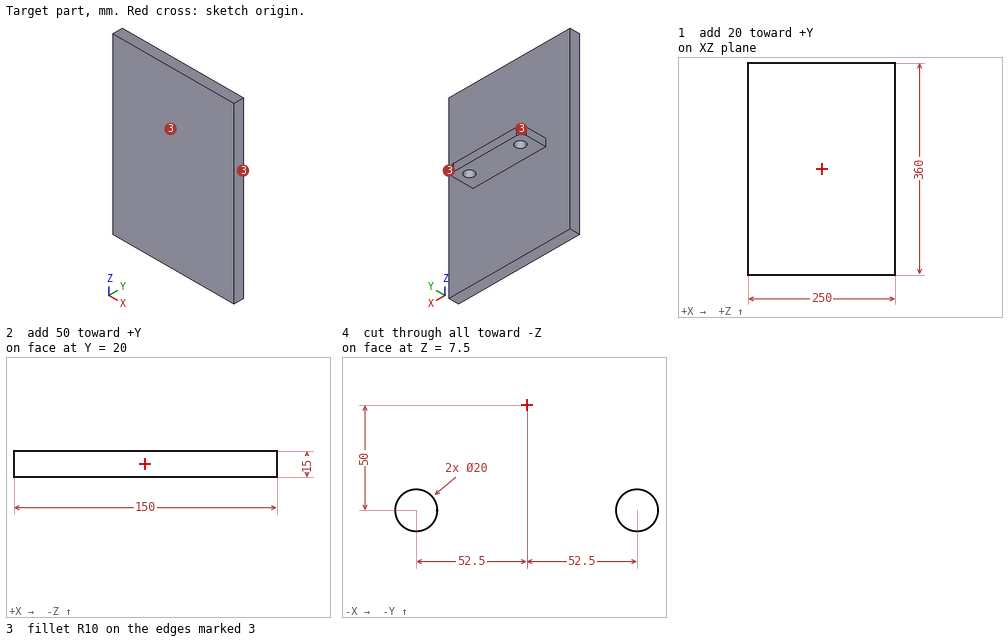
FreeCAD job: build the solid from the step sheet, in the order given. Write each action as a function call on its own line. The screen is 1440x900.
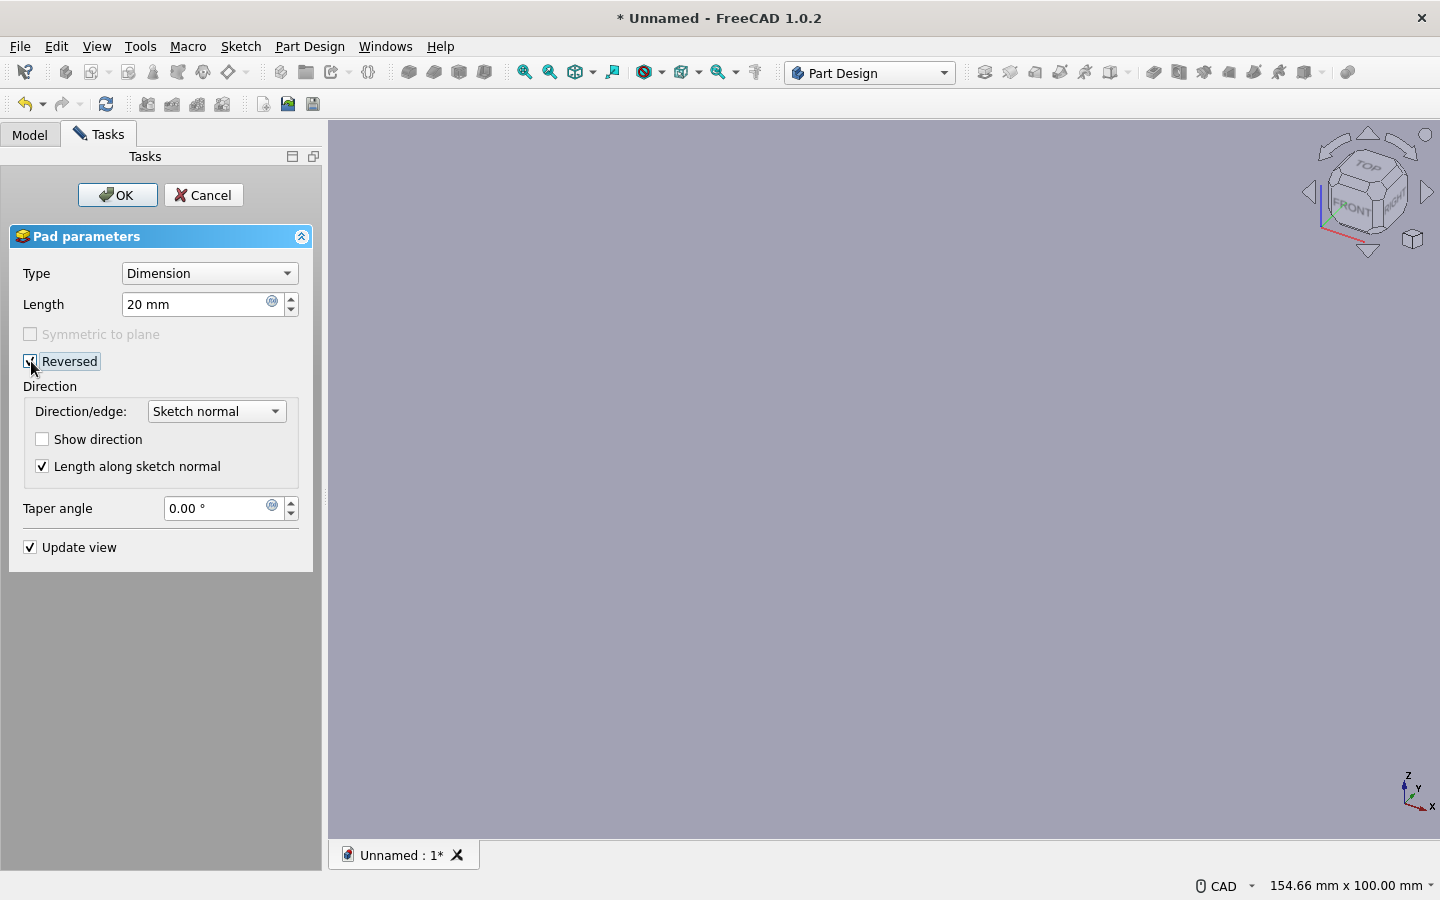
click(118, 195)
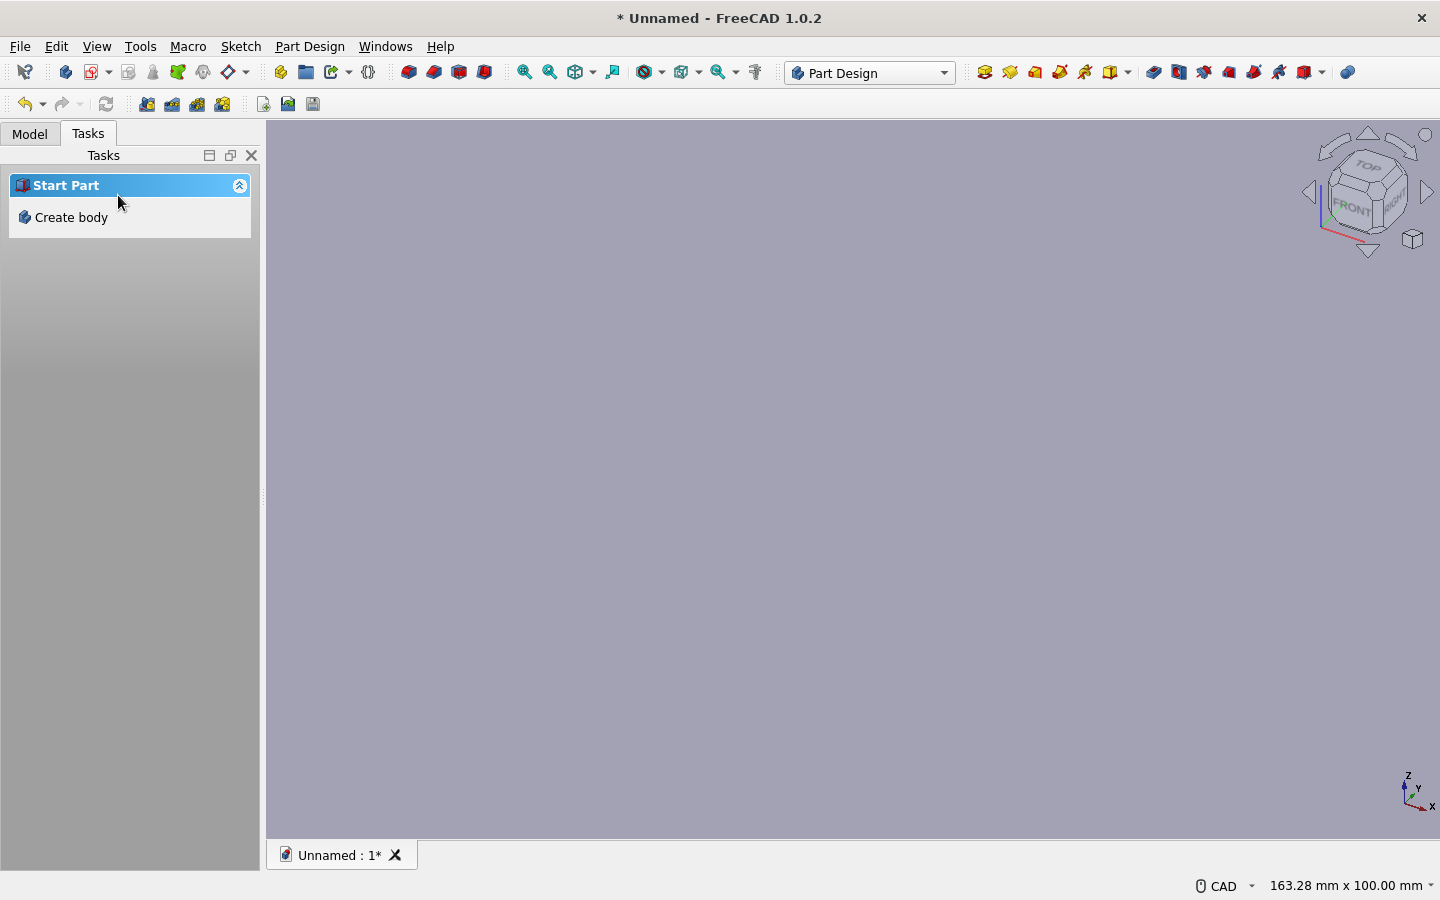
key(v)
key(f)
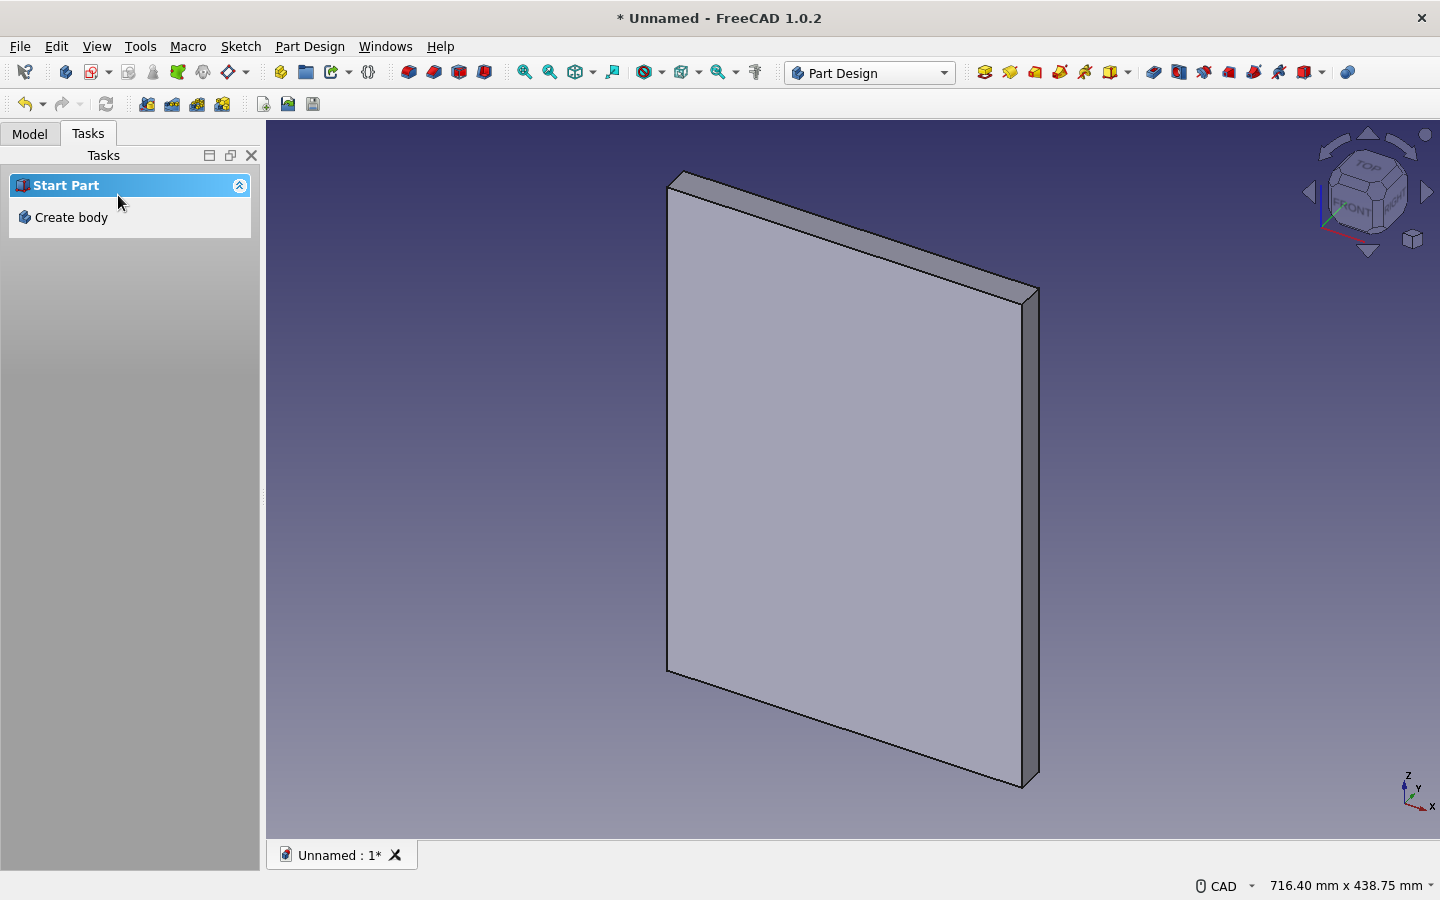
key(4)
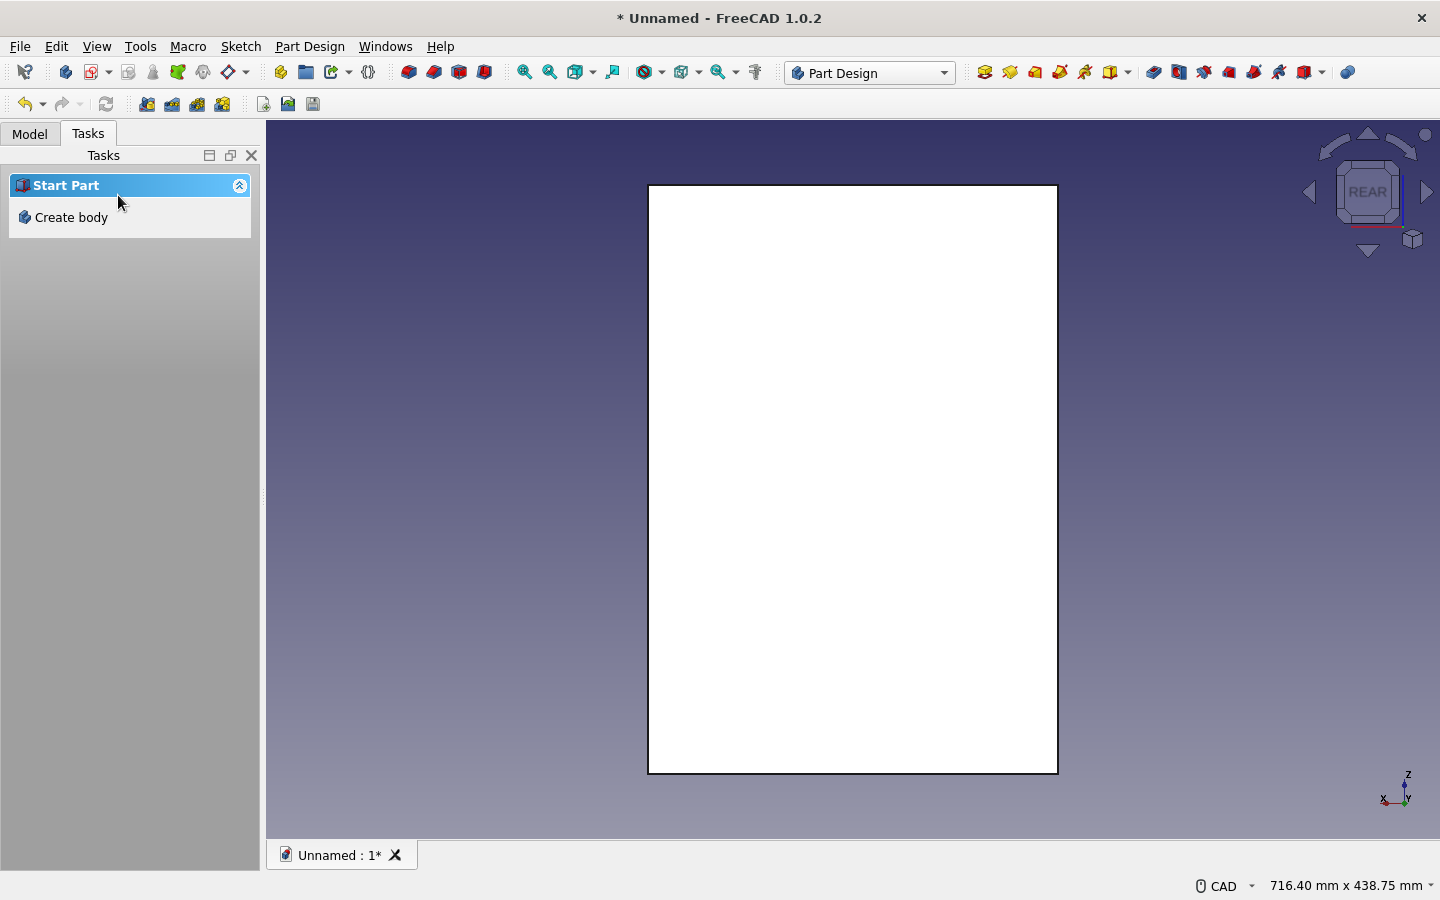
click(853, 394)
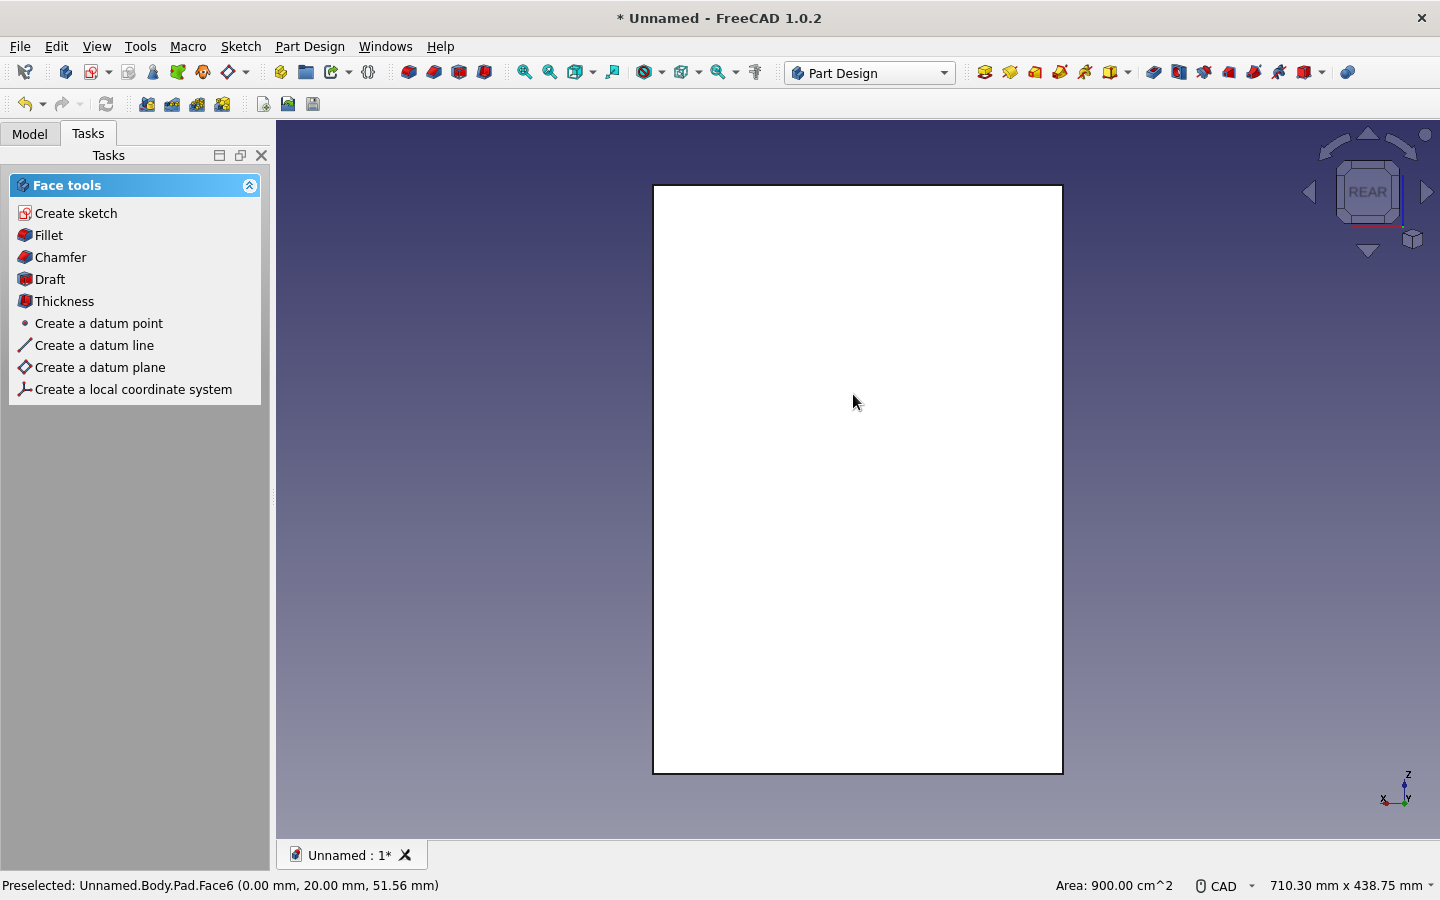
click(90, 72)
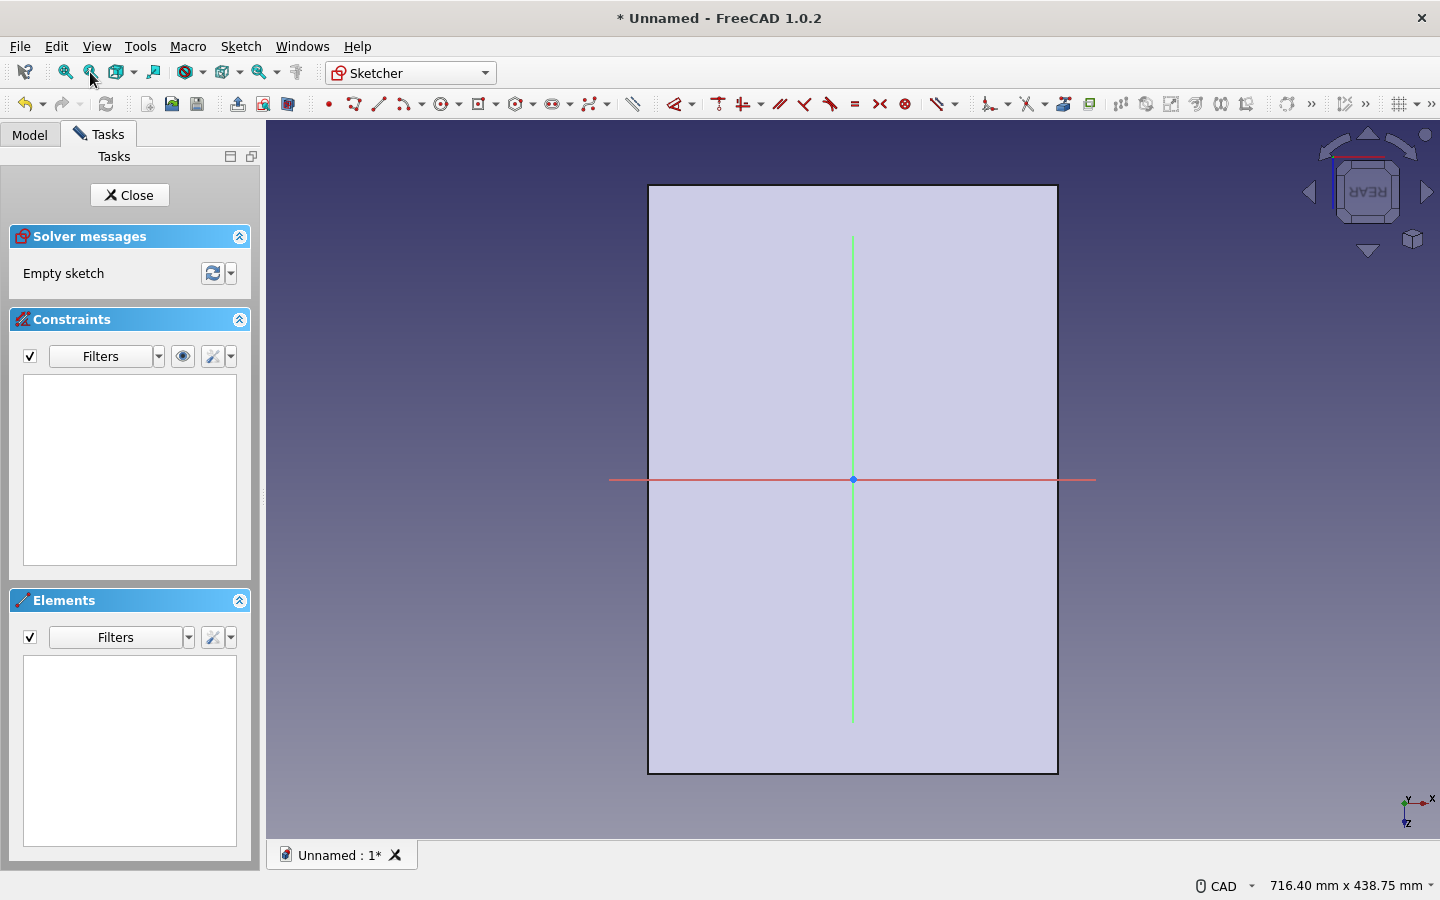
scroll(893, 479, up, 5)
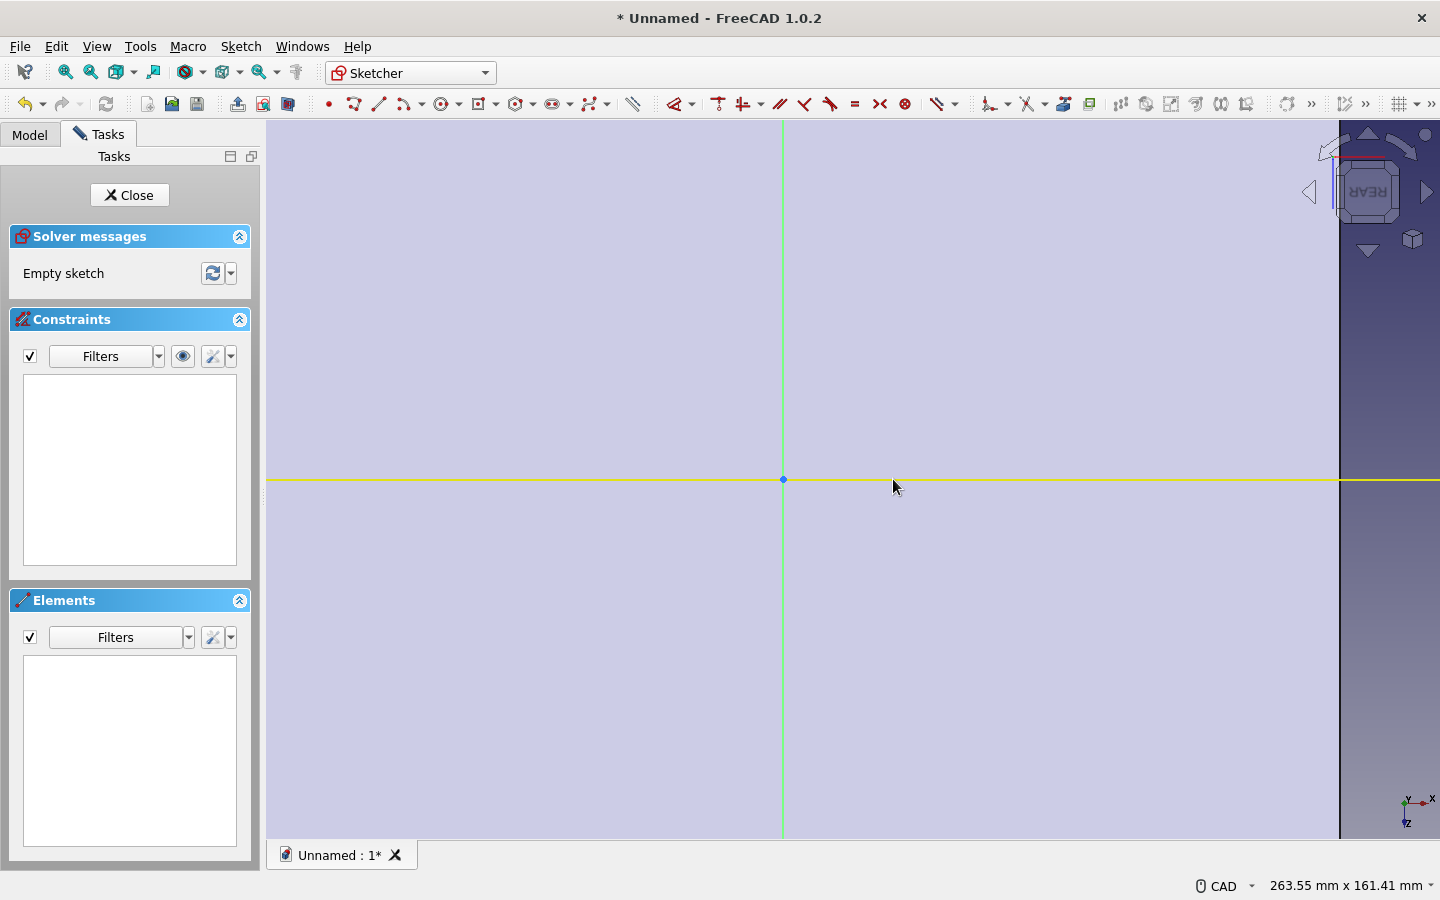
click(478, 104)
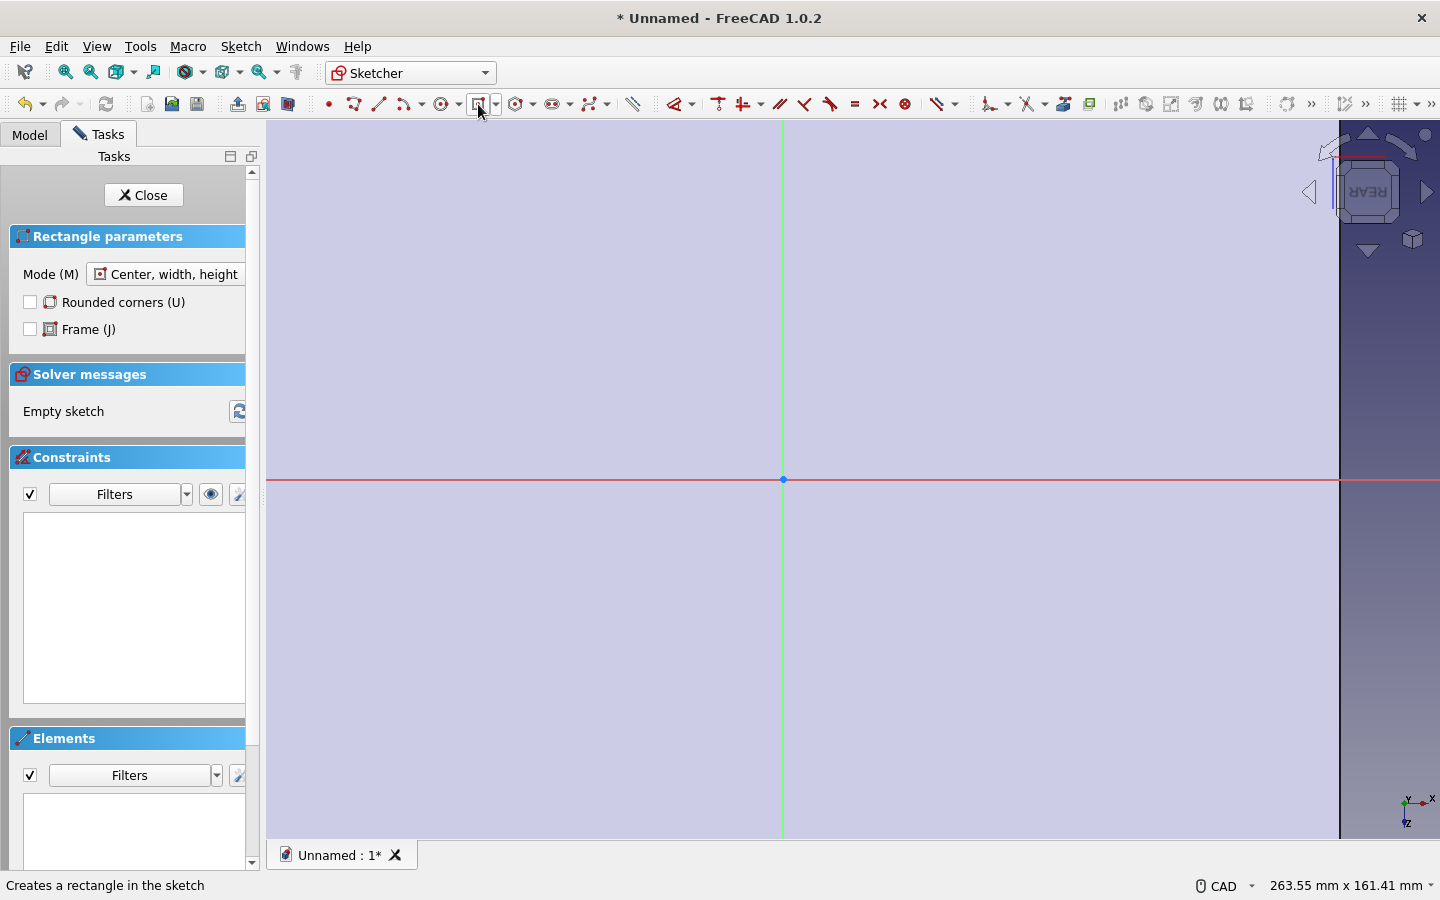
click(783, 479)
click(1117, 446)
key(Escape)